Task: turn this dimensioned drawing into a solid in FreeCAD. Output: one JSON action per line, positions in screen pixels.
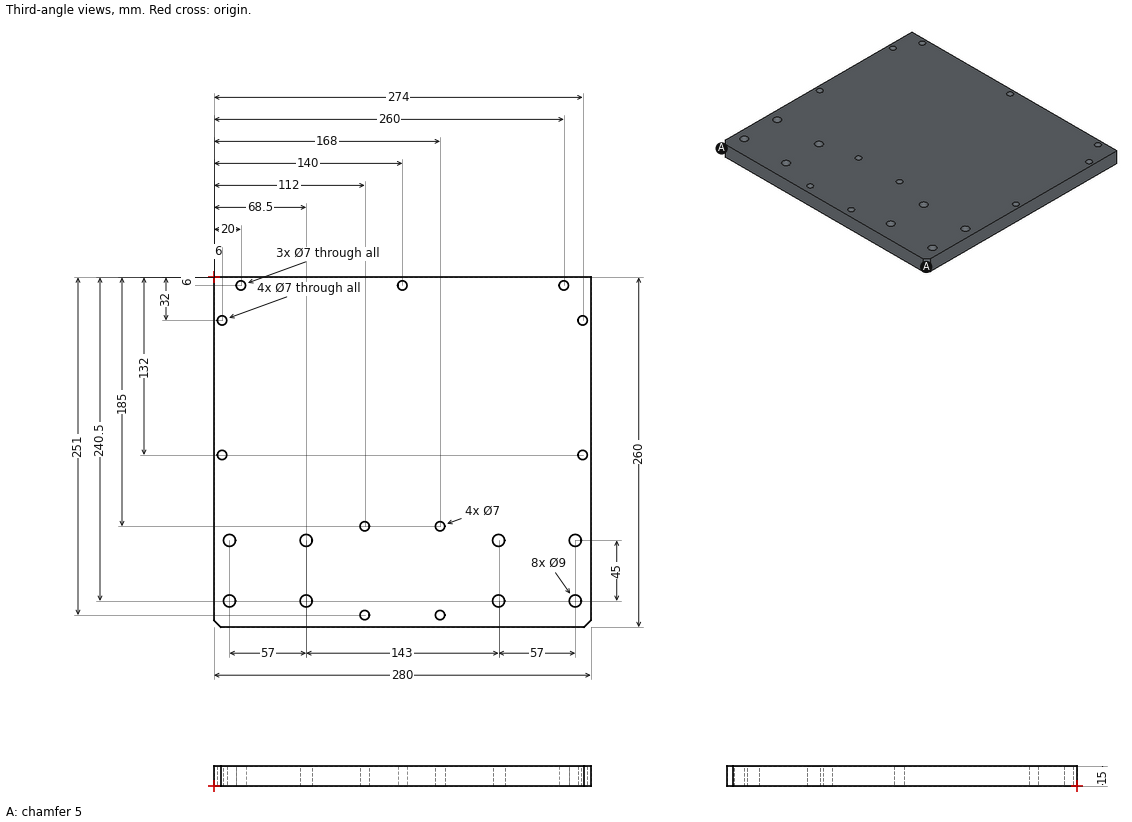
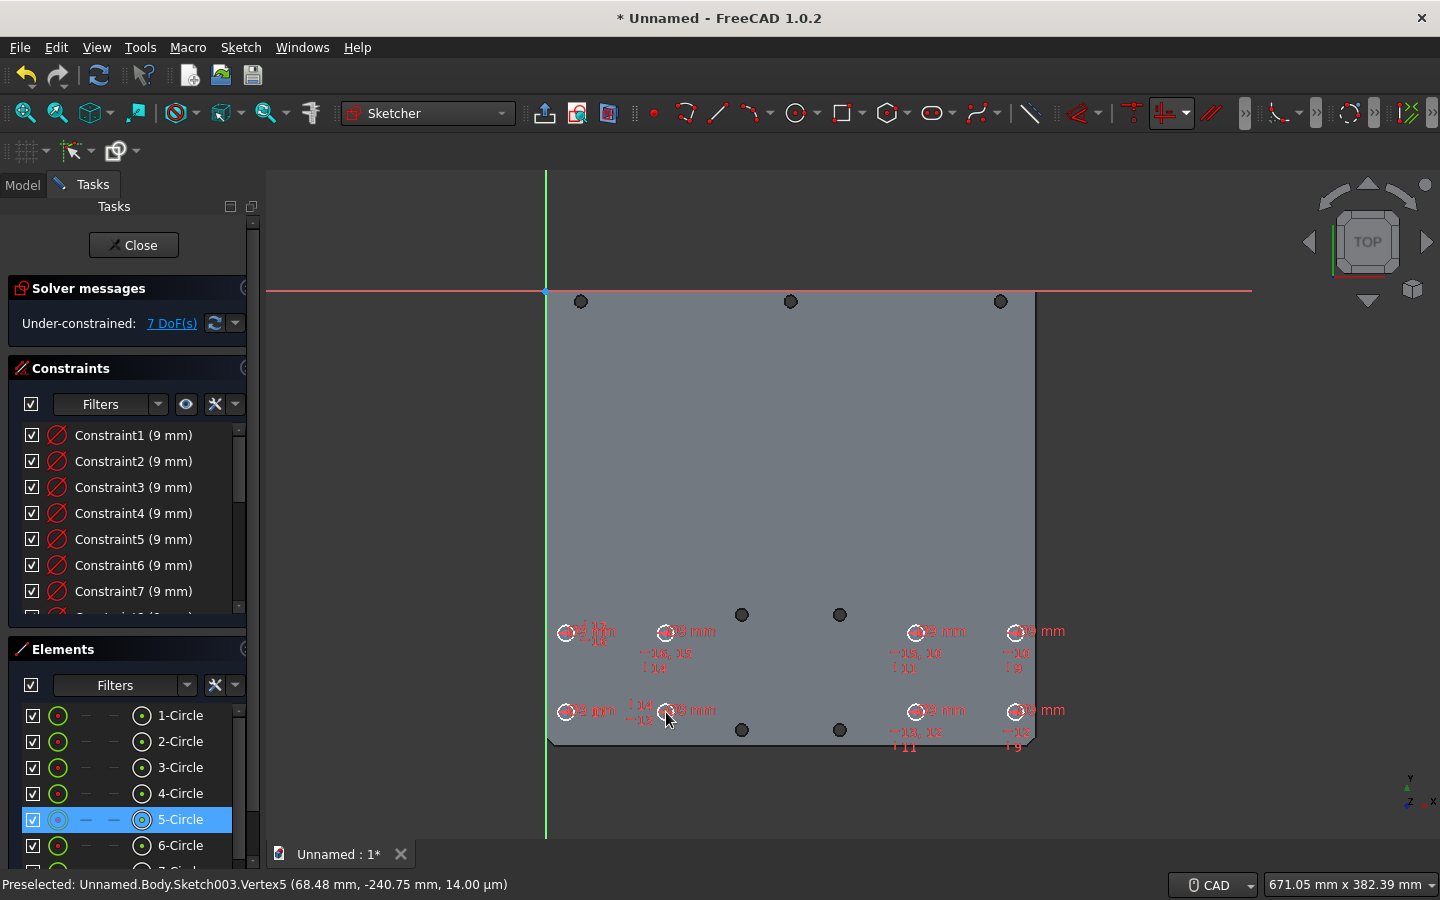
{"action": "left_click", "coordinate": [566, 712]}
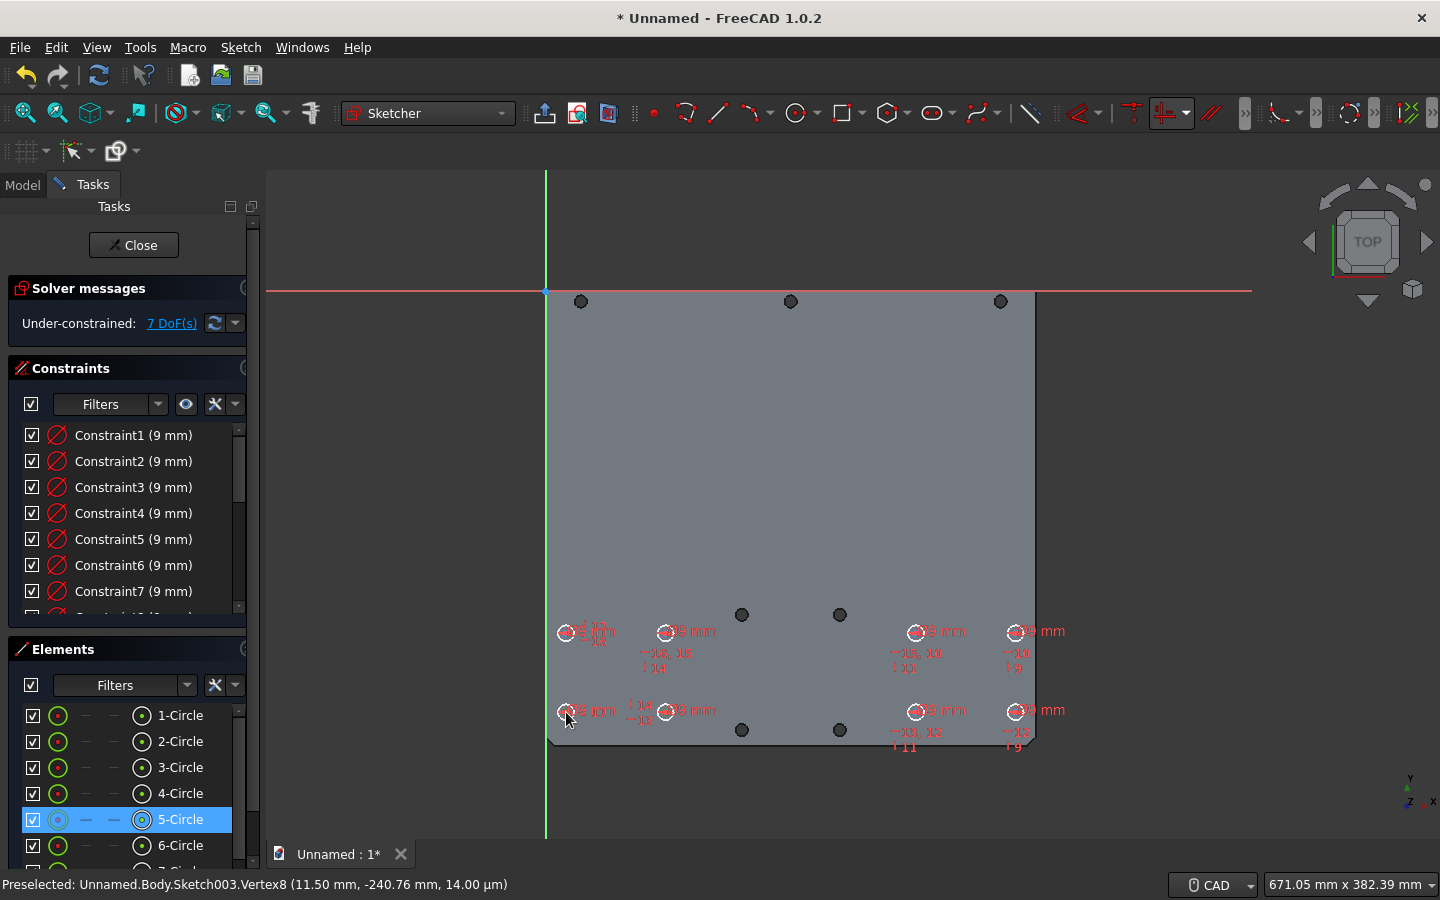
{"action": "left_click", "coordinate": [1188, 114]}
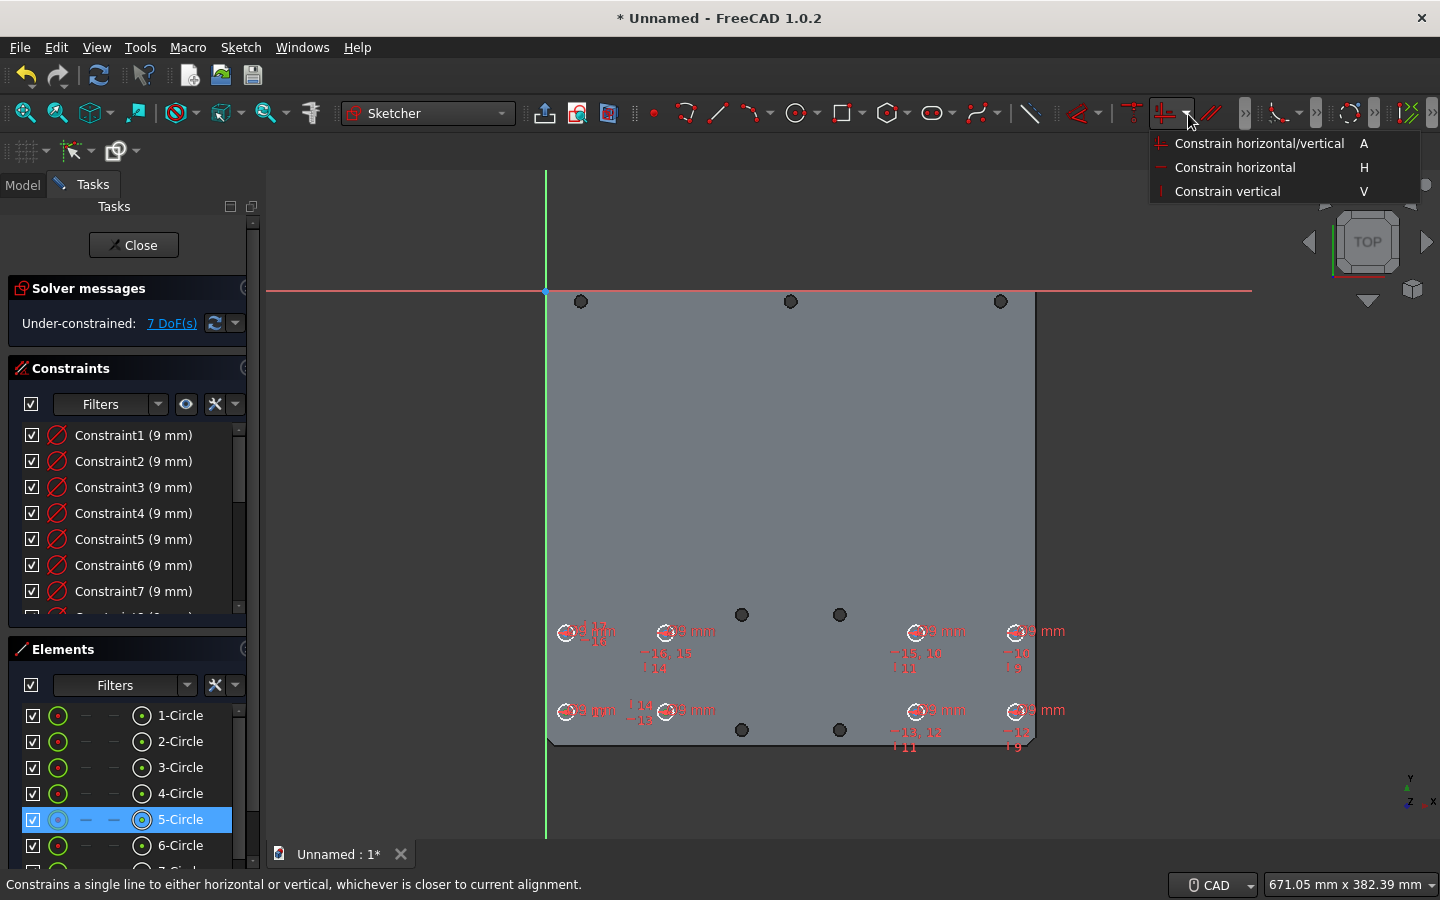
{"action": "left_click", "coordinate": [1285, 167]}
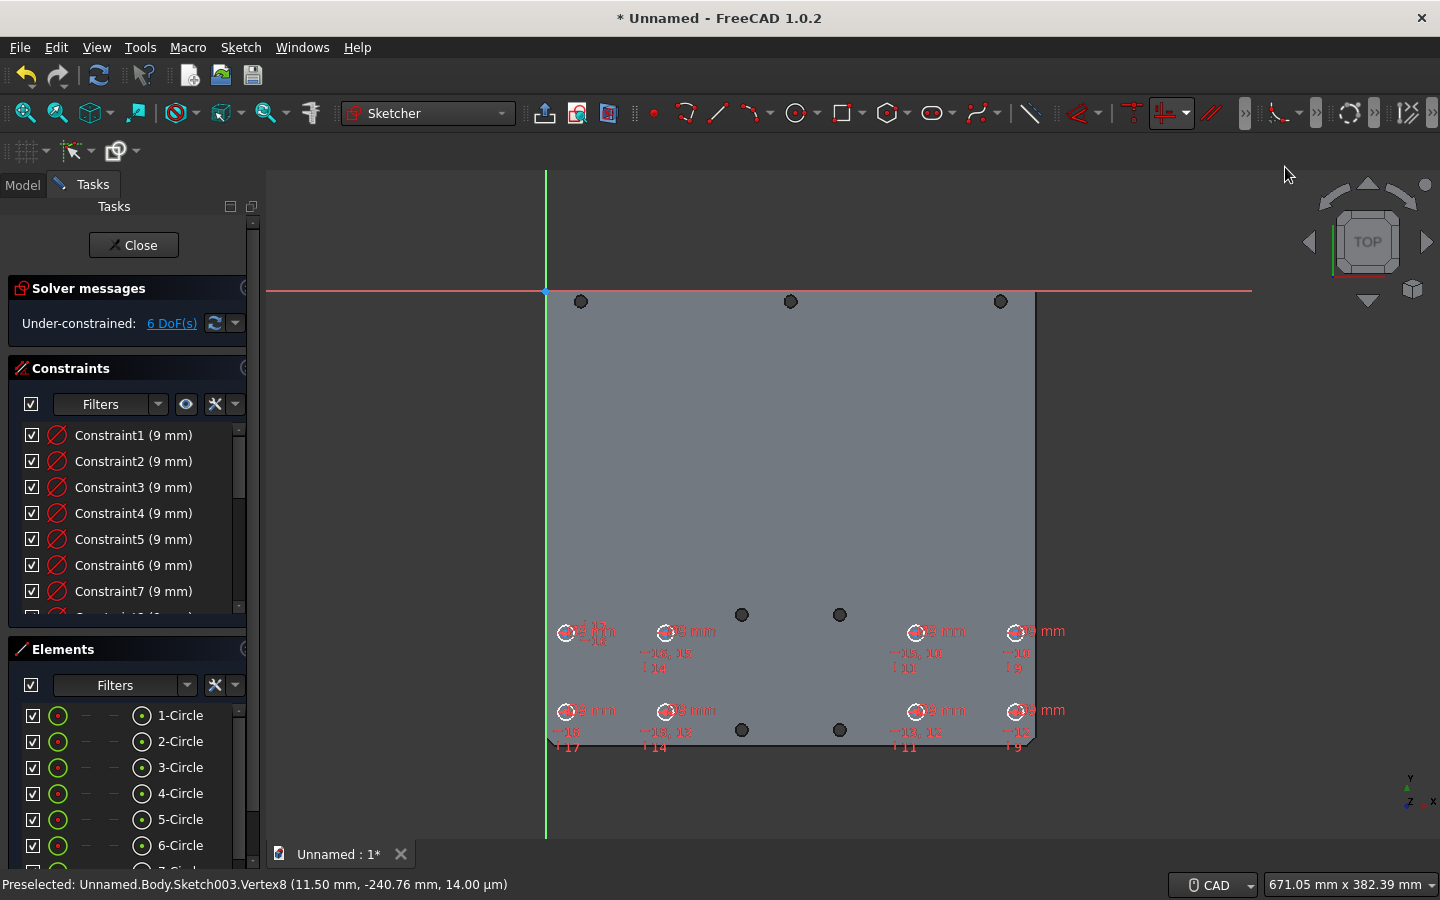
{"action": "left_click", "coordinate": [1078, 114]}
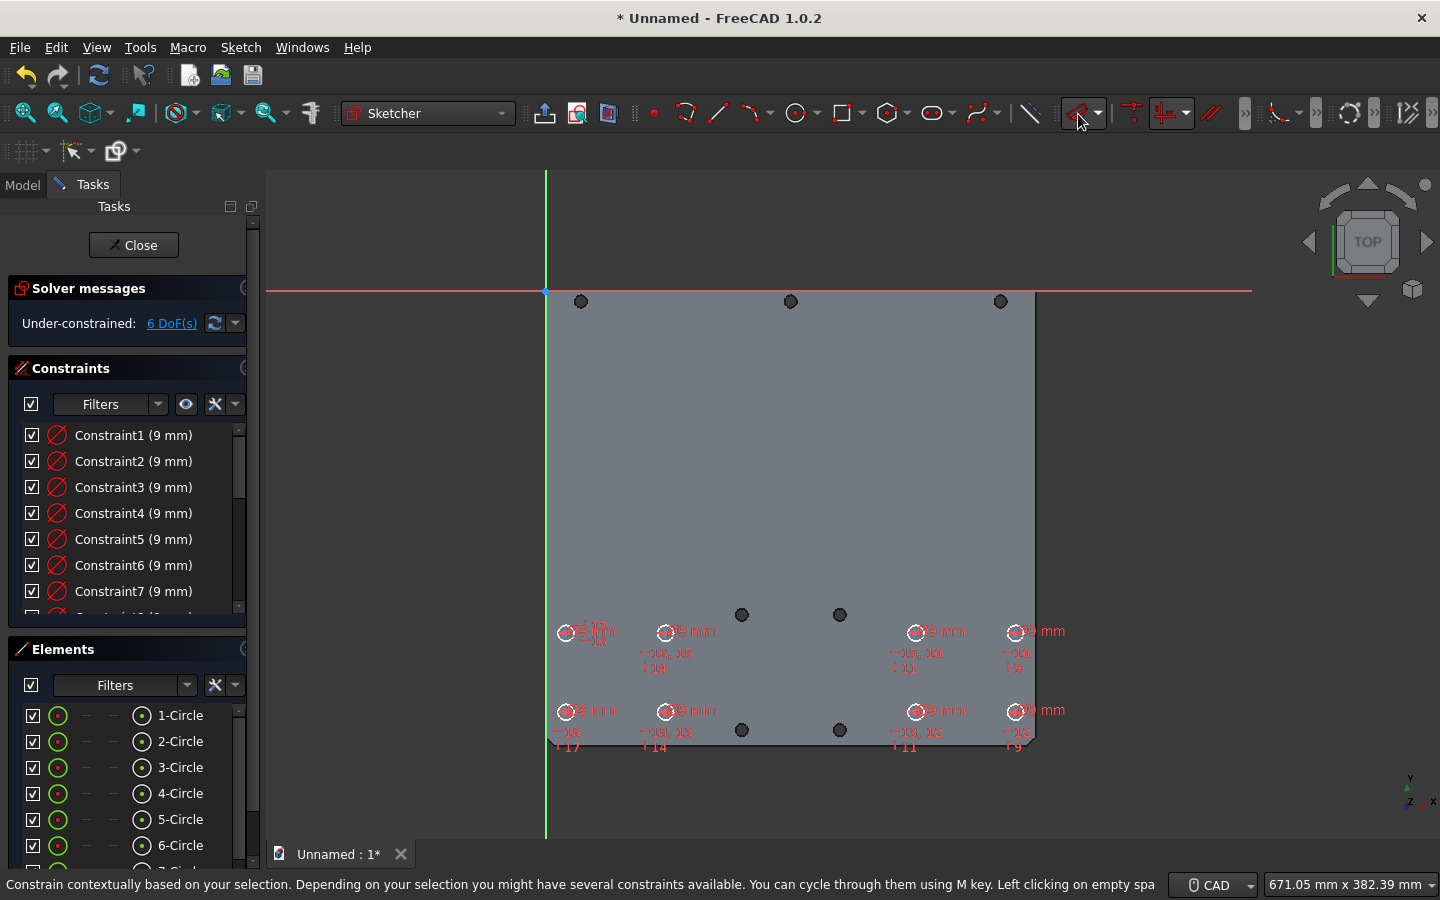
{"action": "left_click", "coordinate": [1016, 712]}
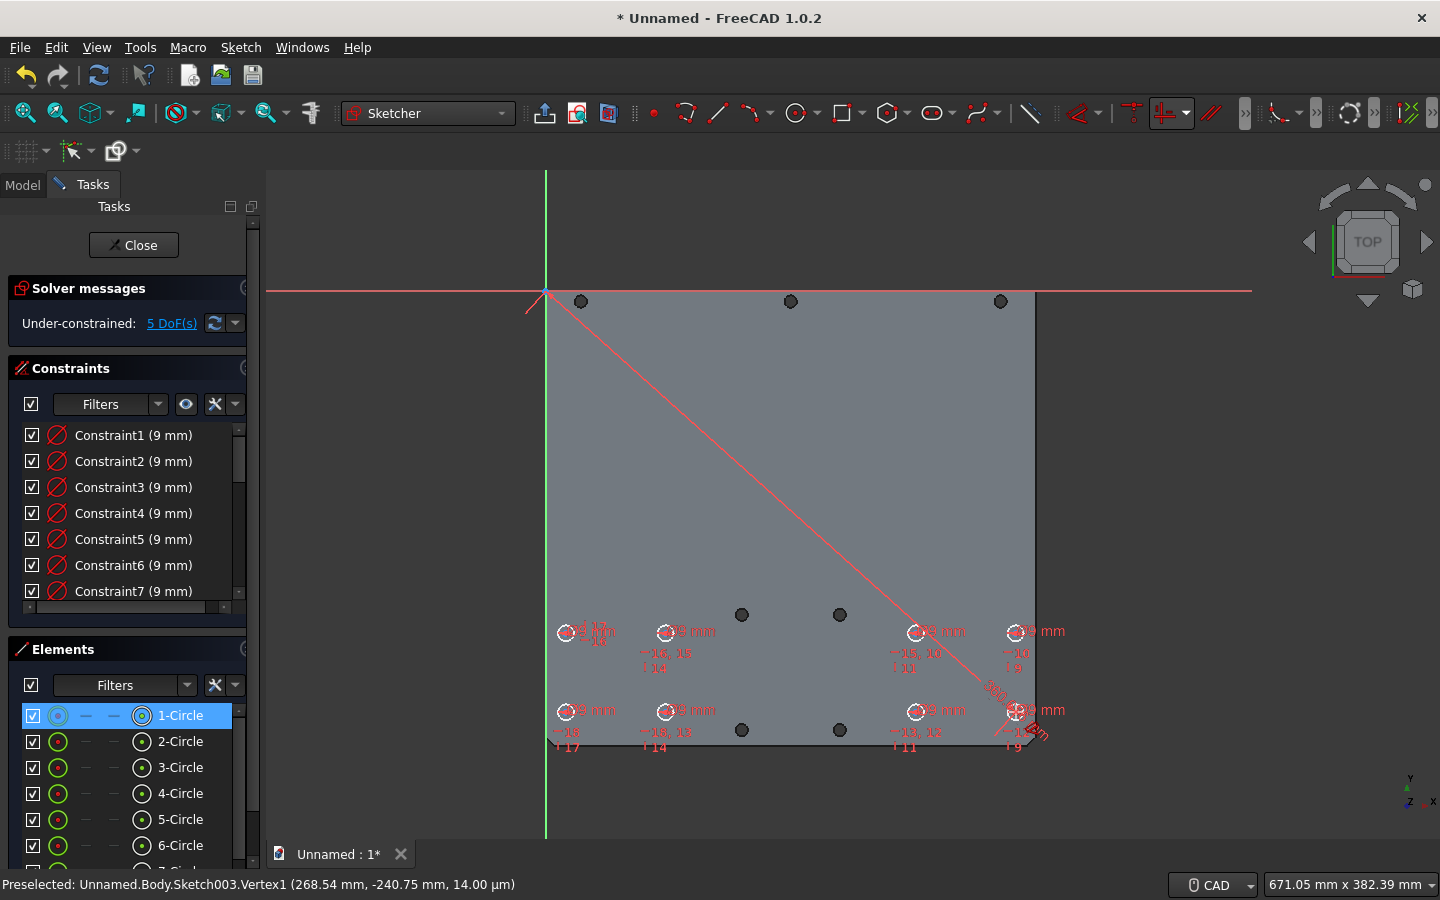
{"action": "left_click", "coordinate": [1016, 633]}
{"action": "left_click", "coordinate": [1050, 673]}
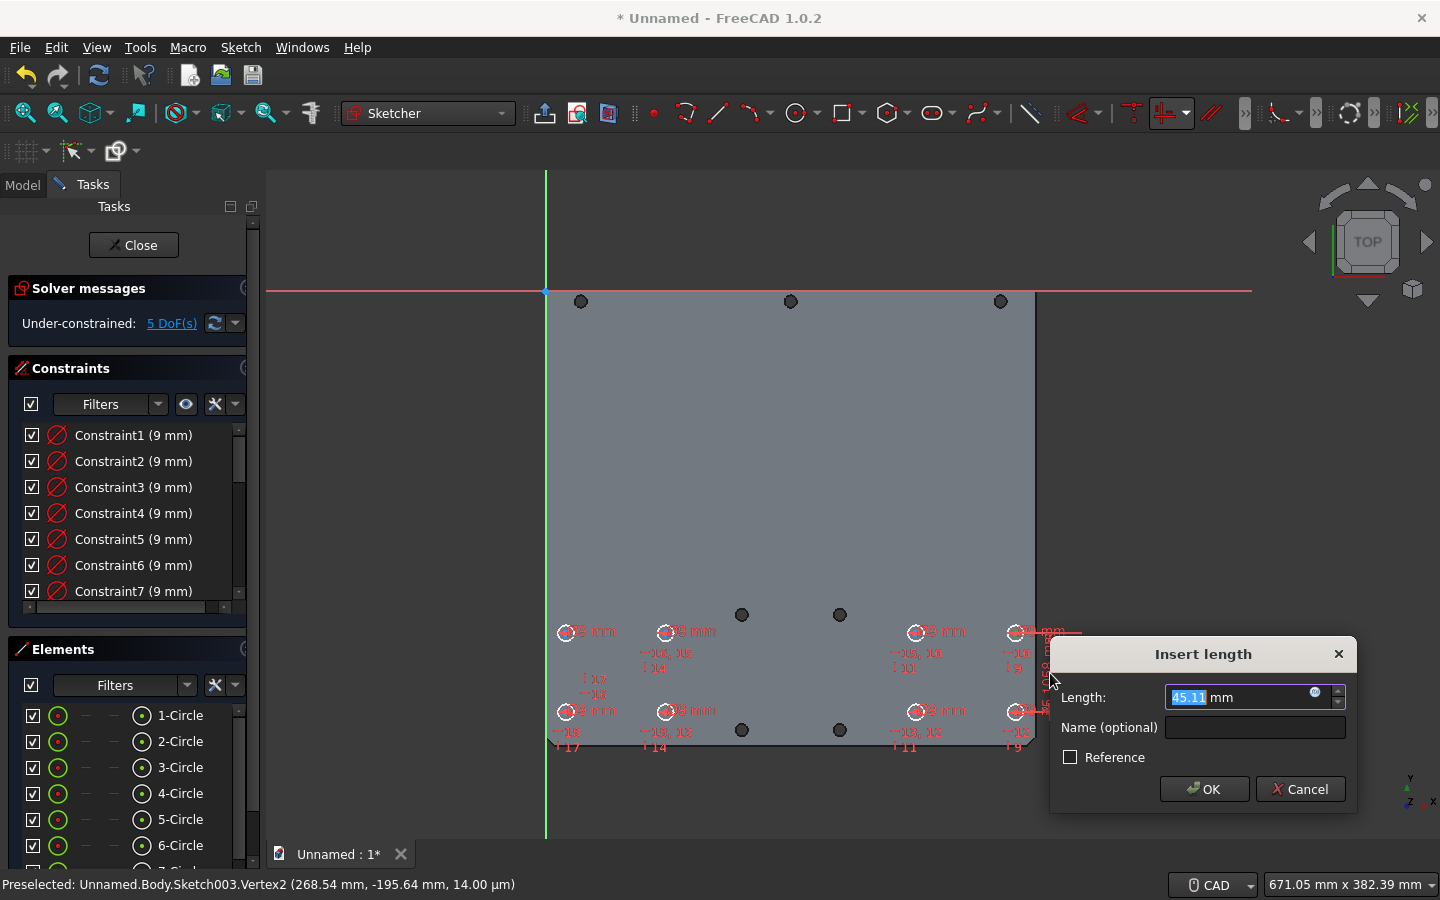
{"action": "type", "text": "45"}
{"action": "key", "text": "Return"}